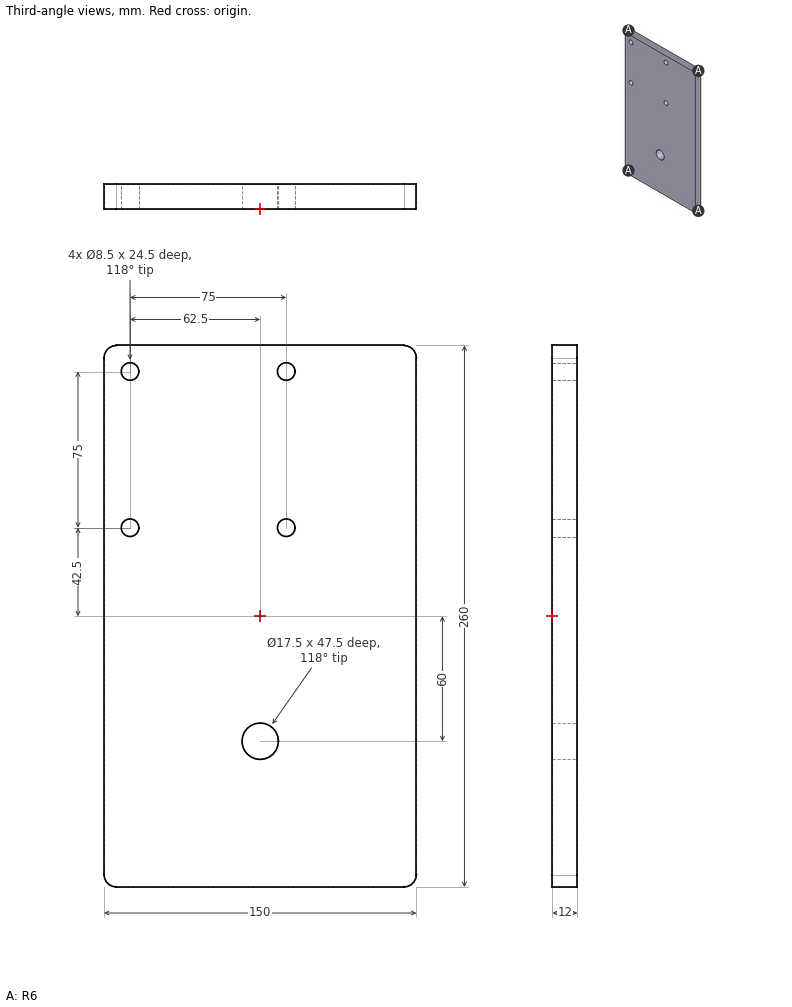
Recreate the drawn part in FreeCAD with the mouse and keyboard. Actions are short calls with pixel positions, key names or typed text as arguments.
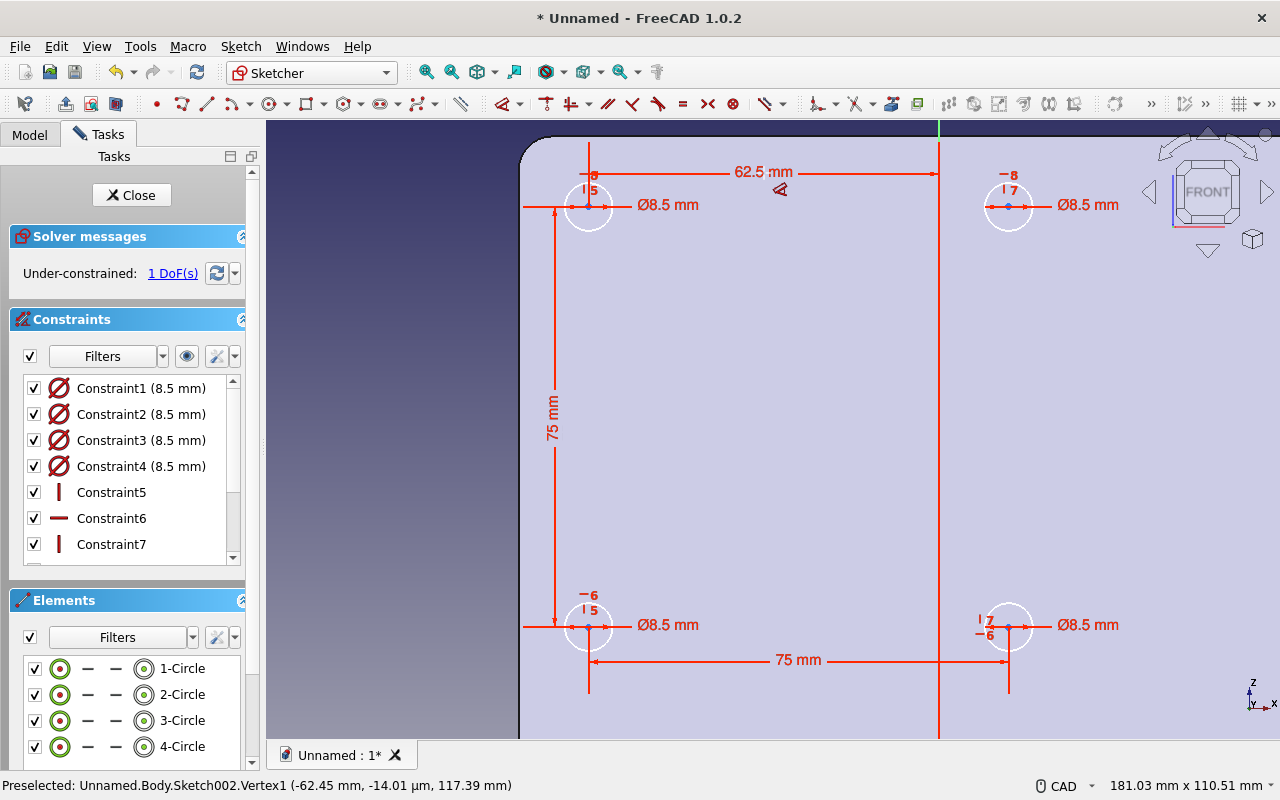
click(589, 627)
click(555, 669)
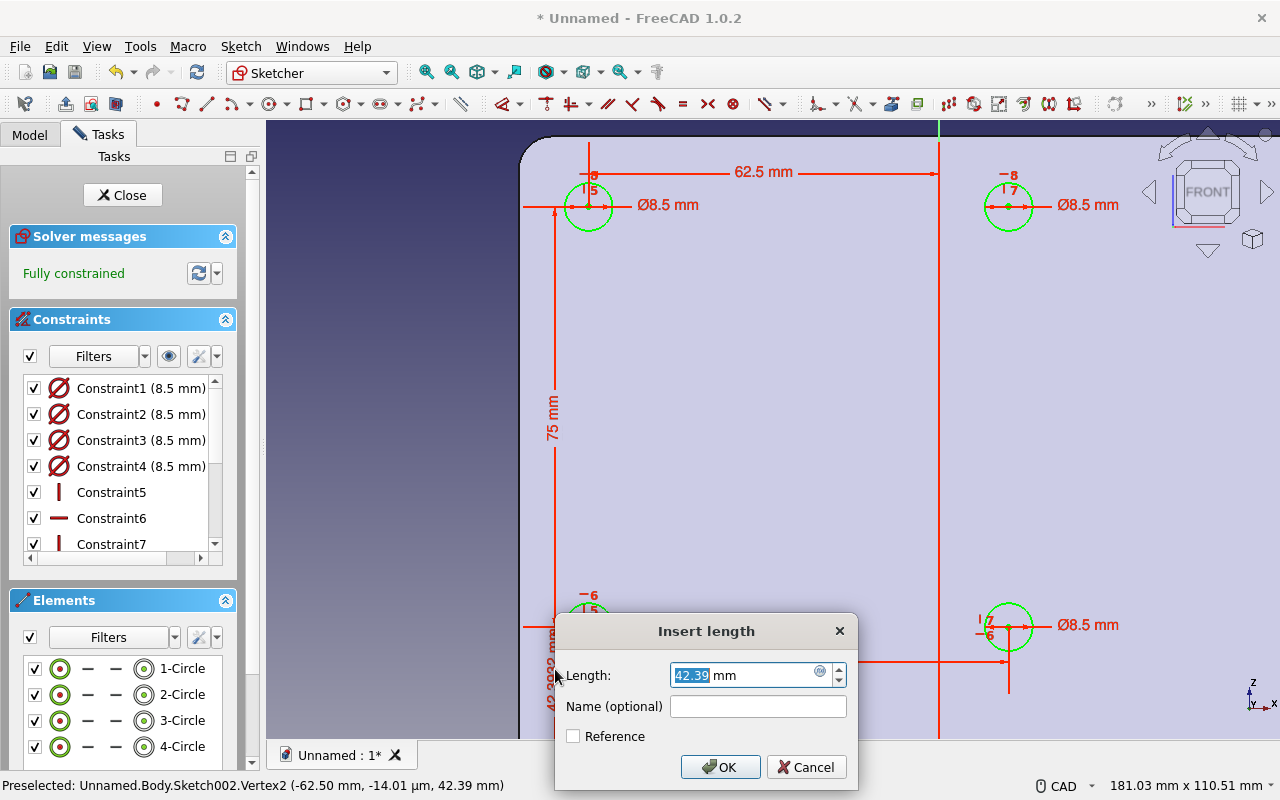
text(42.5)
key(Return)
key(Escape)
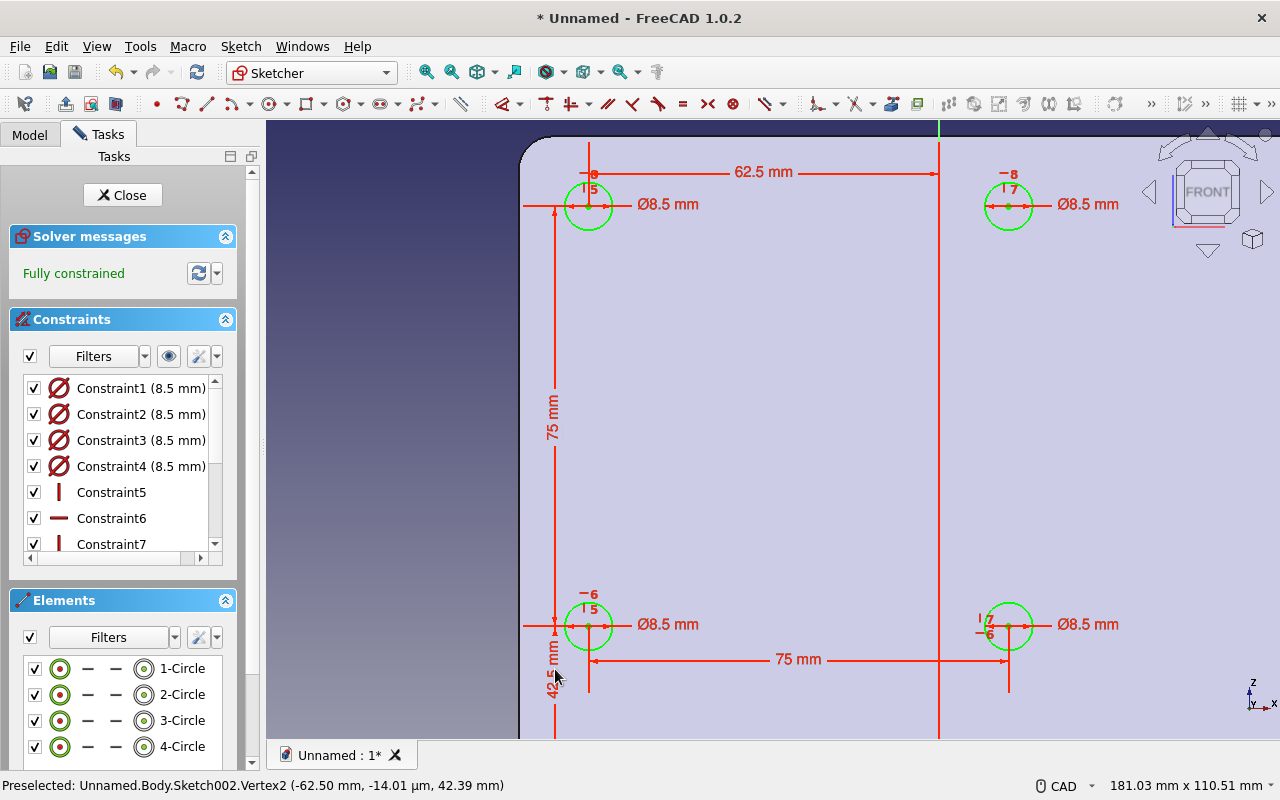
click(123, 195)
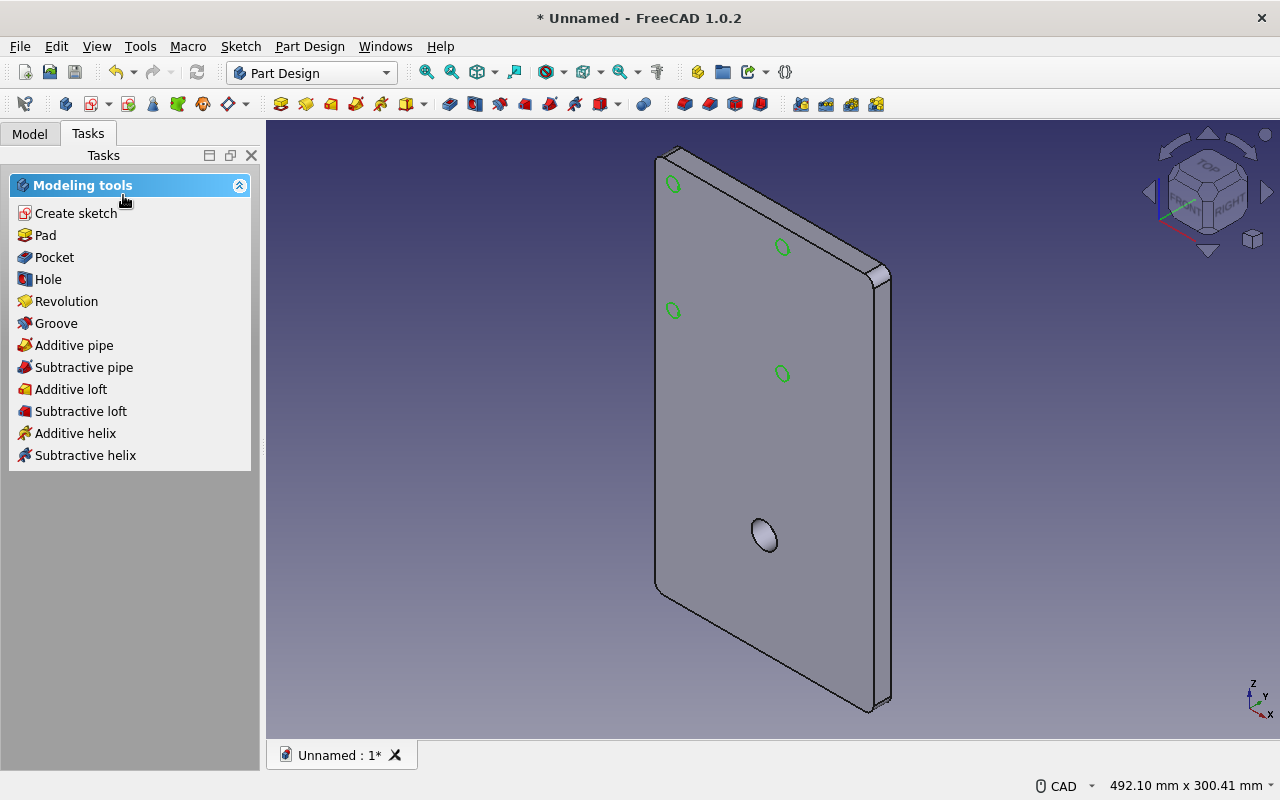
click(475, 104)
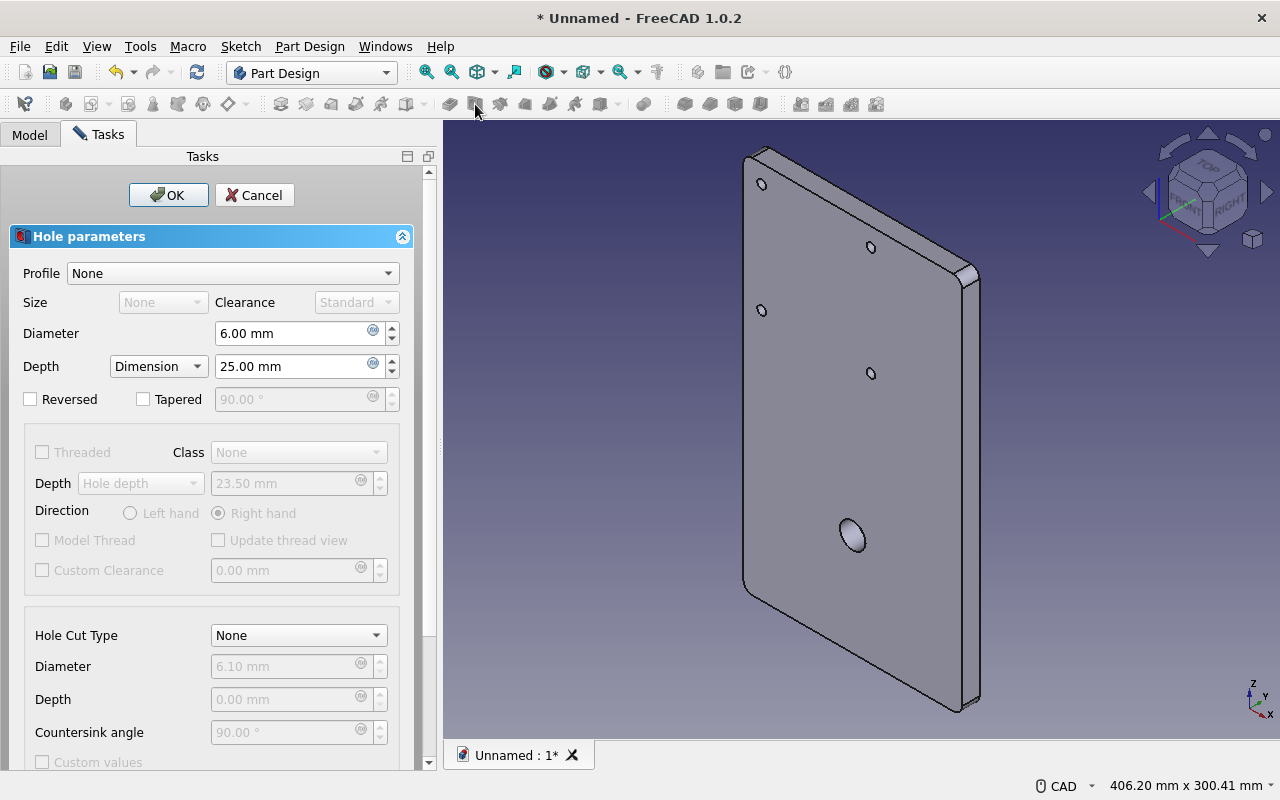
triple_click(300, 334)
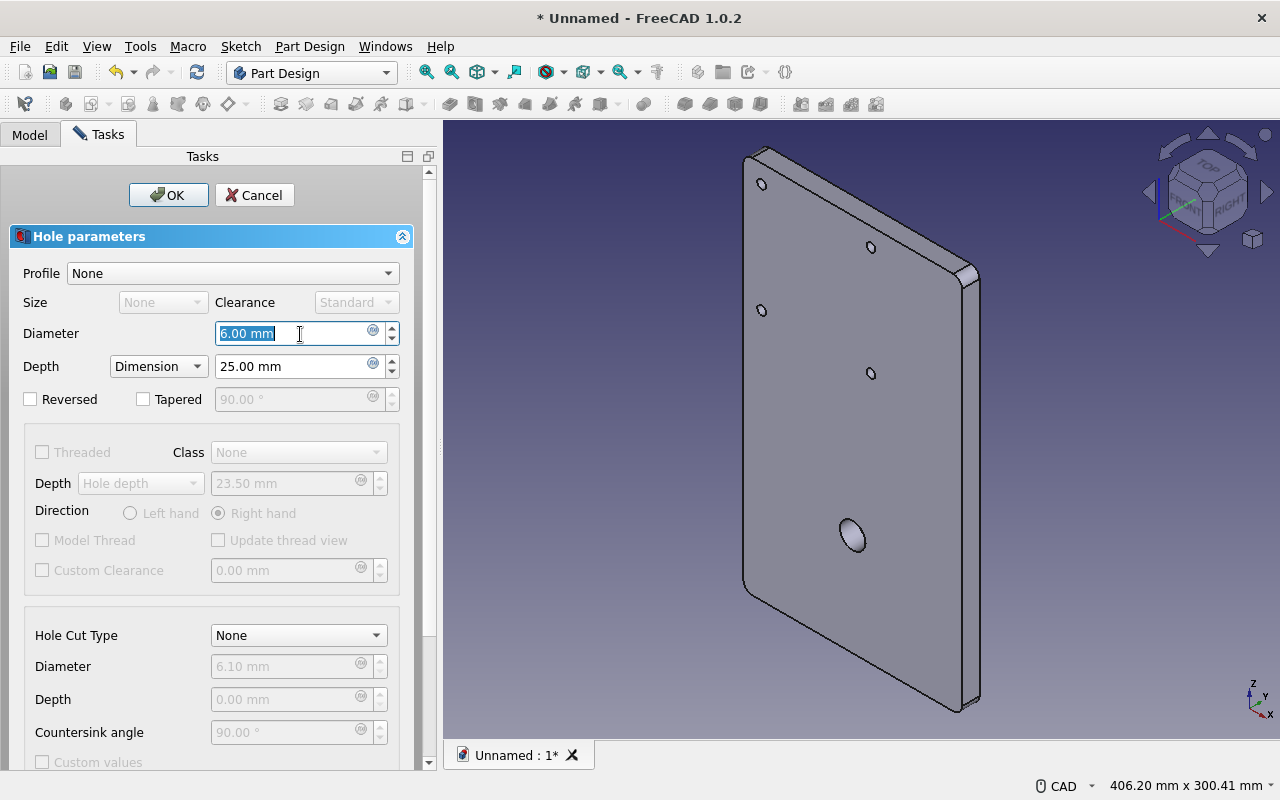
text(8.5)
key(Tab)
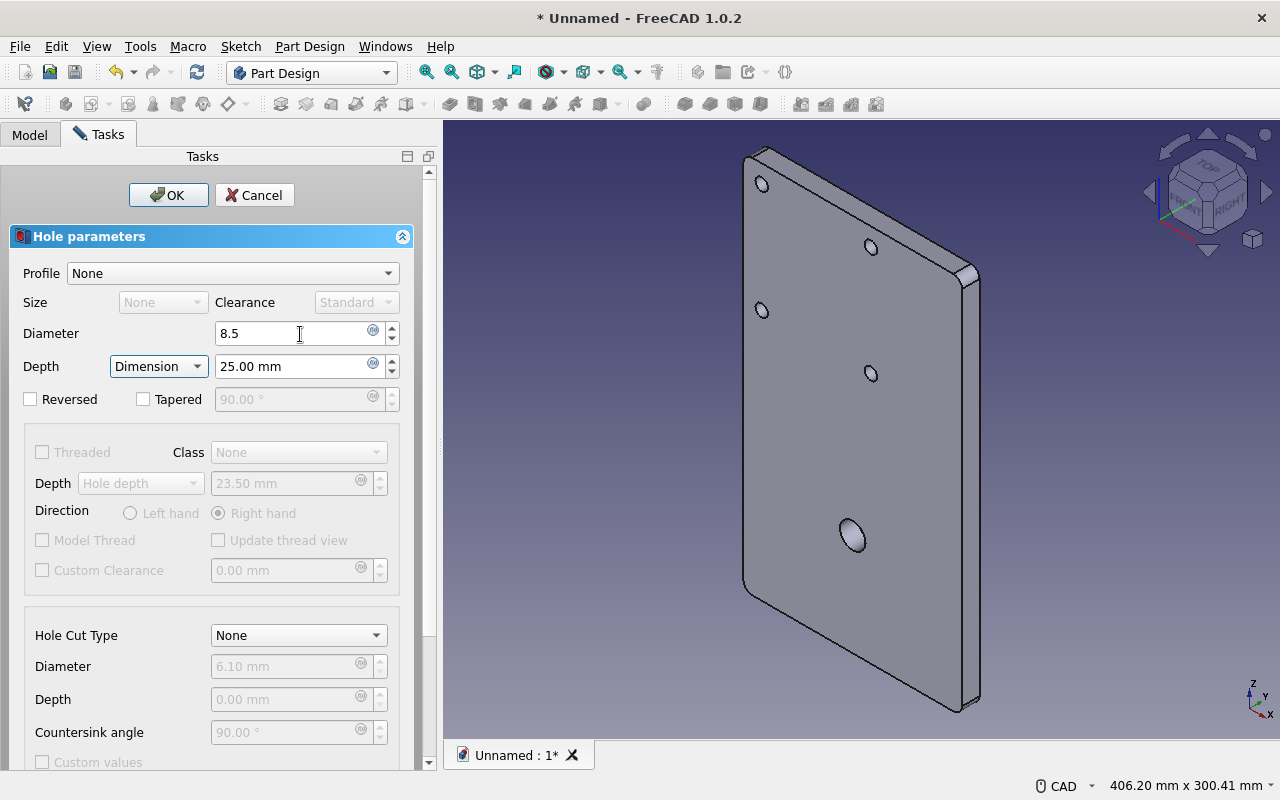
triple_click(300, 366)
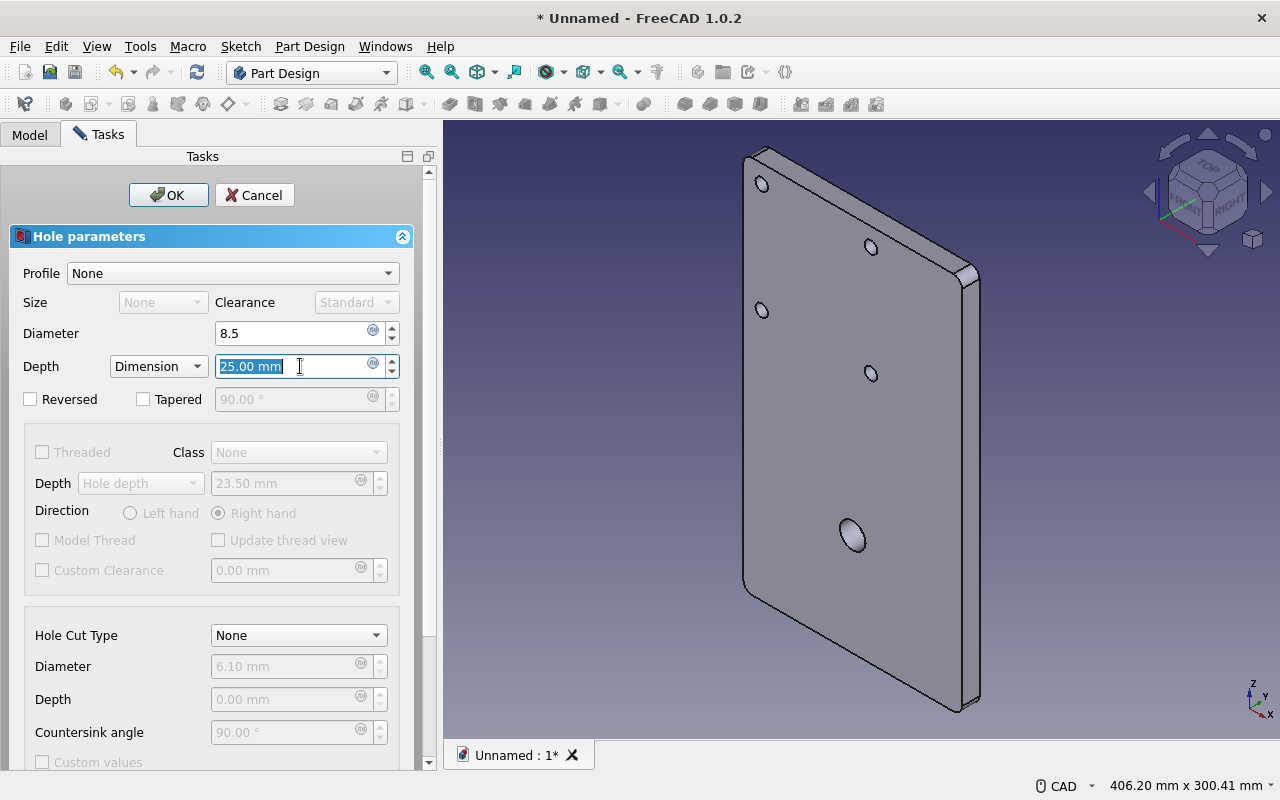
text(24.5)
key(Tab)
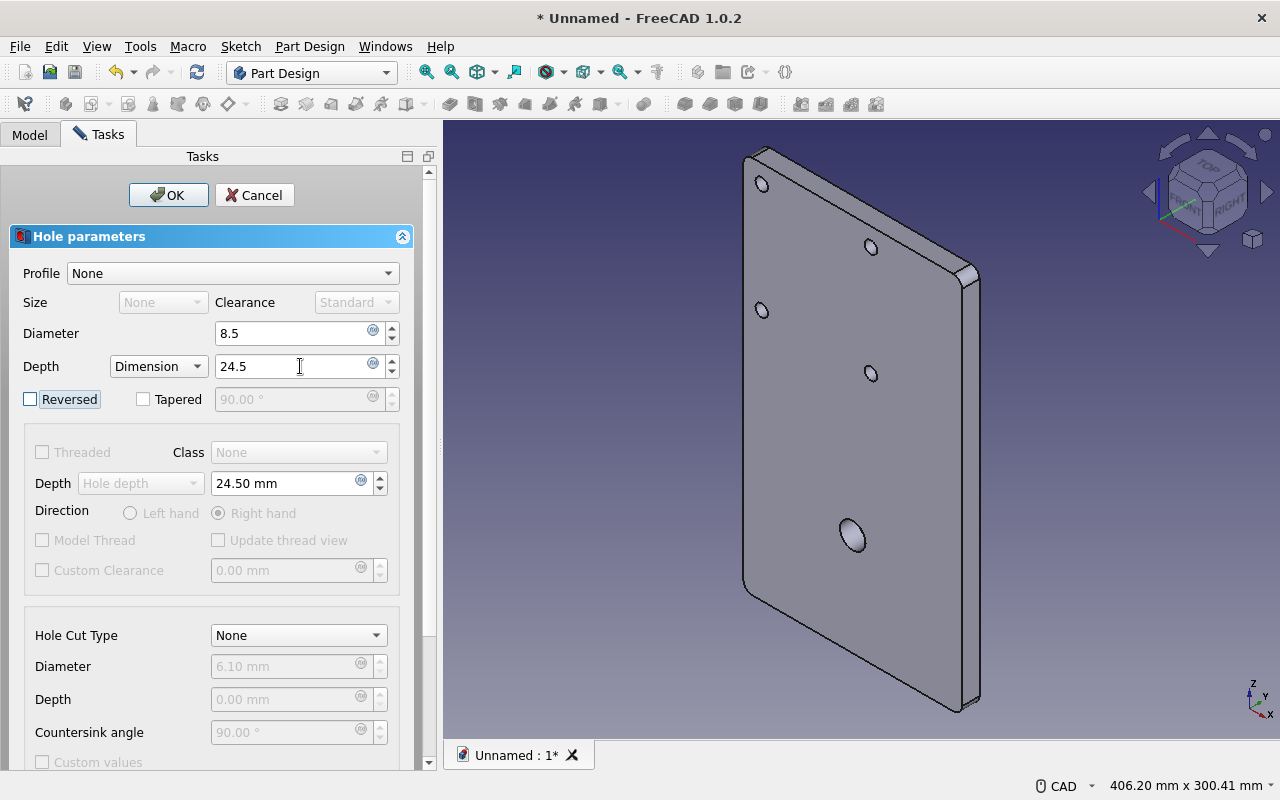
click(169, 195)